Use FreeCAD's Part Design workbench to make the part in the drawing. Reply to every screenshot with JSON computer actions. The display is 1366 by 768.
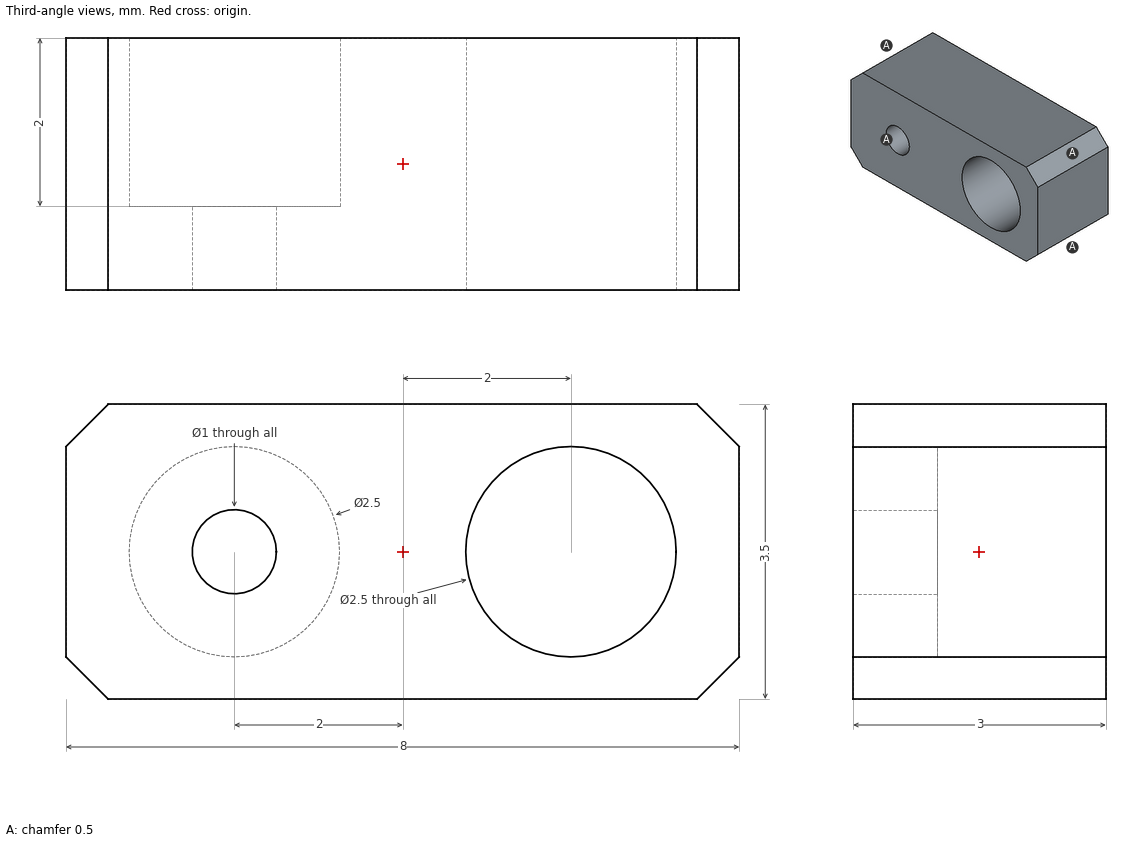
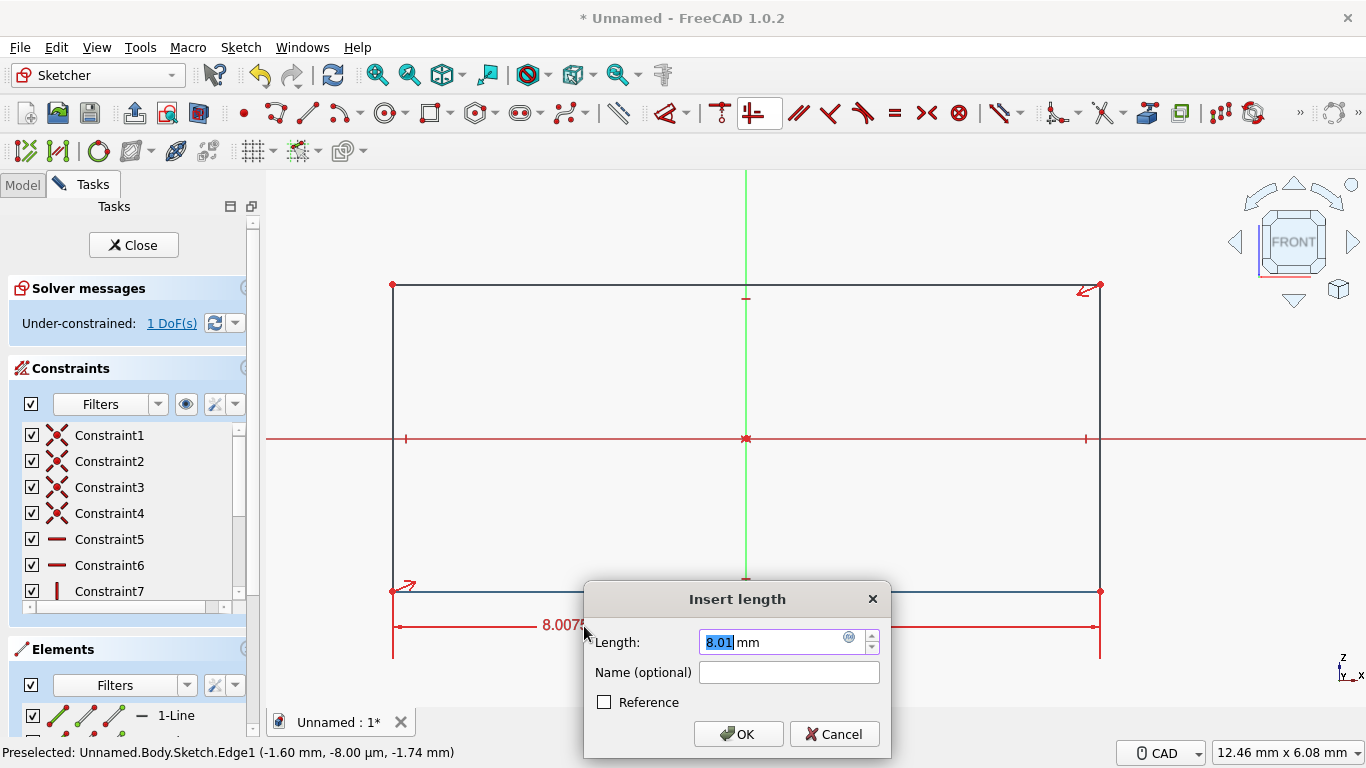
{"action": "type", "text": "8"}
{"action": "key", "text": "Return"}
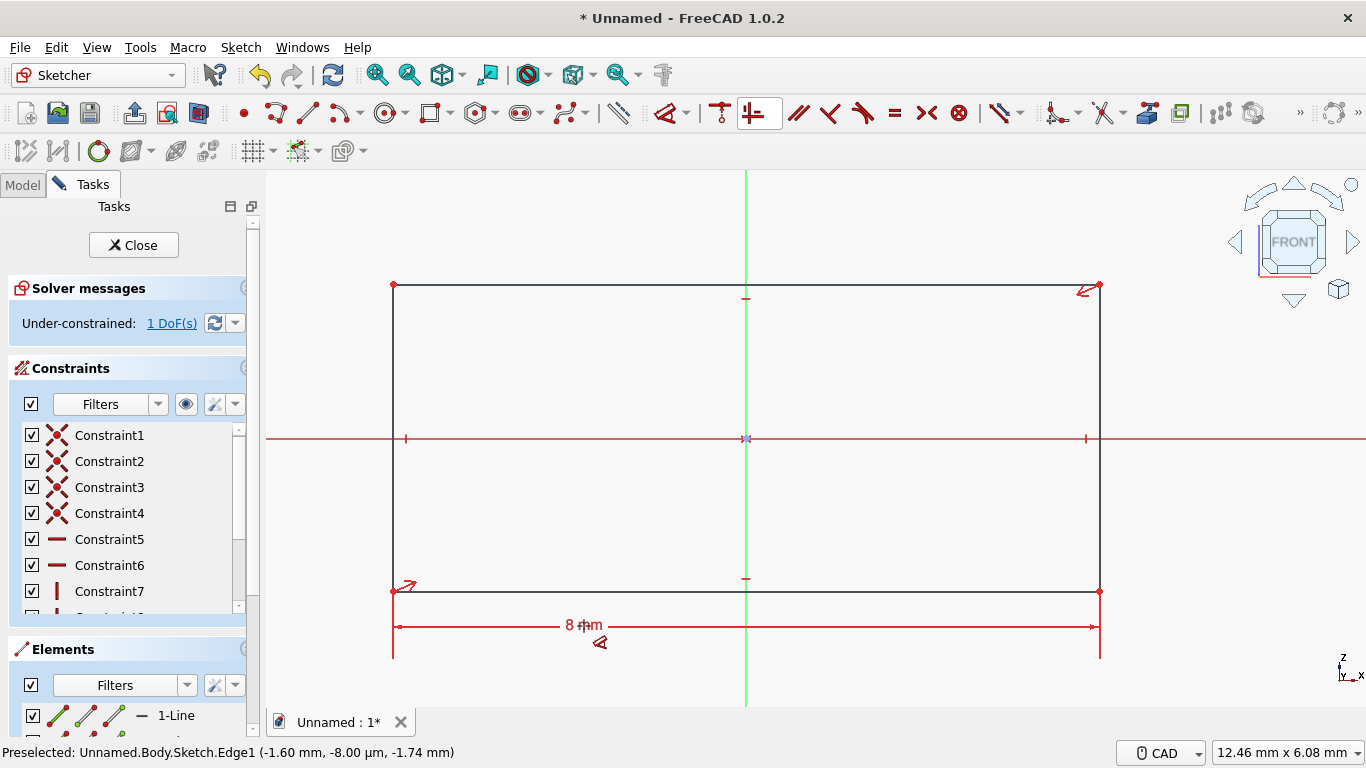
{"action": "left_click", "coordinate": [1100, 500]}
{"action": "left_click", "coordinate": [1134, 368]}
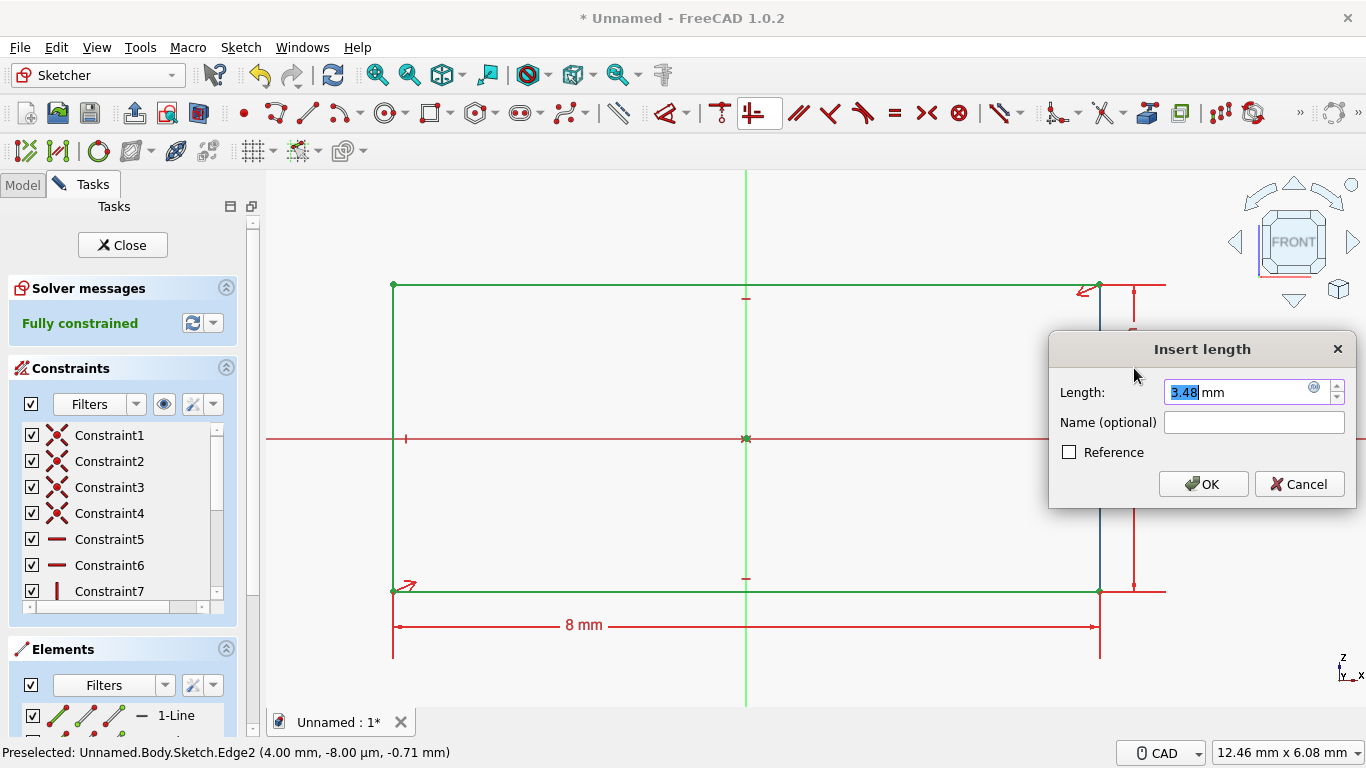
{"action": "type", "text": "3.5"}
{"action": "key", "text": "Return"}
{"action": "key", "text": "Escape"}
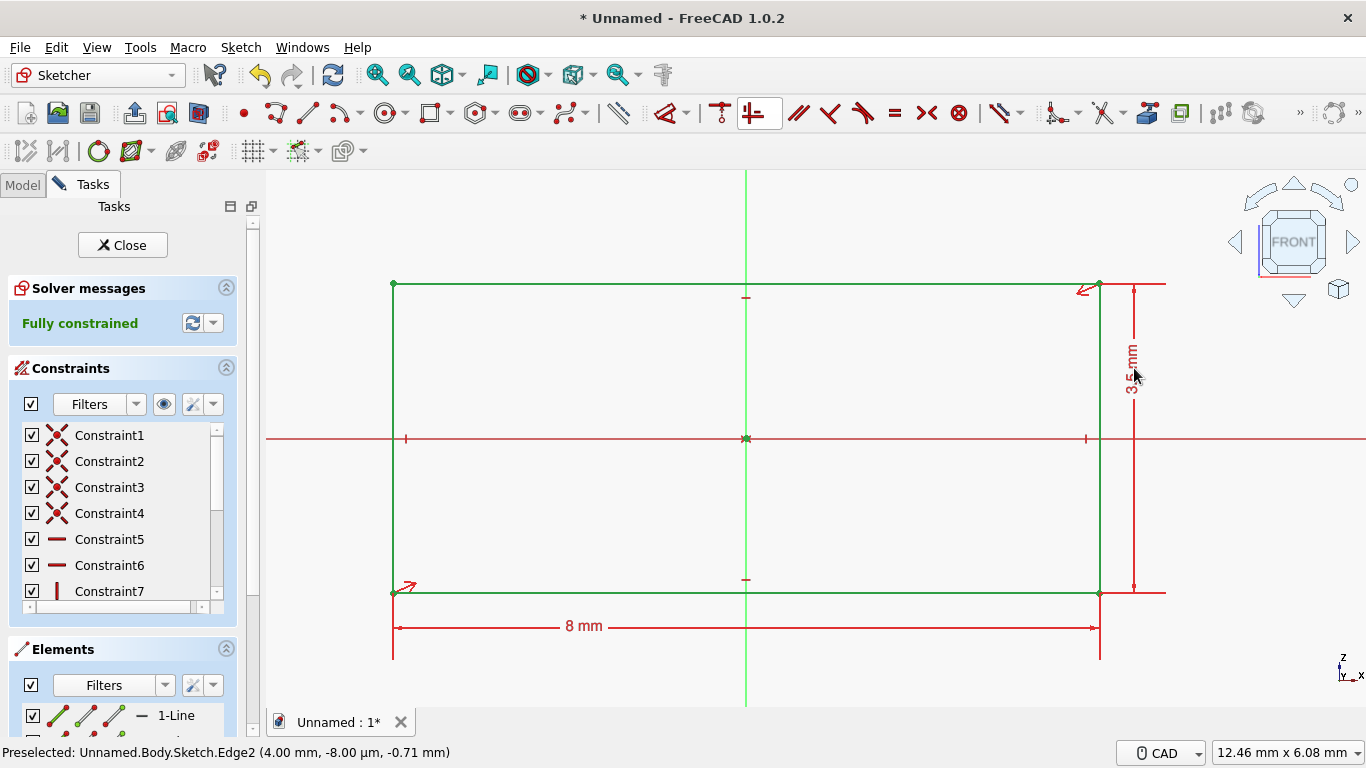
{"action": "left_click", "coordinate": [123, 245]}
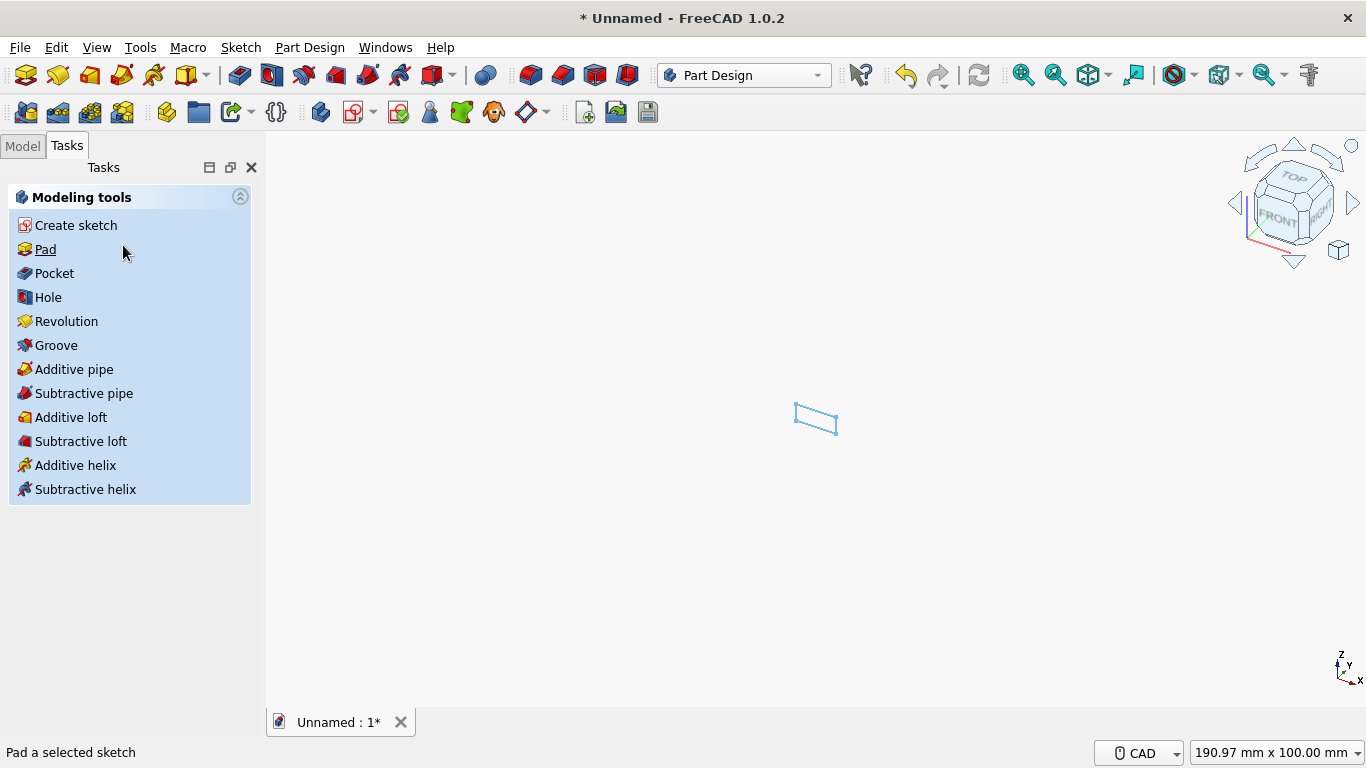
{"action": "left_click", "coordinate": [26, 76]}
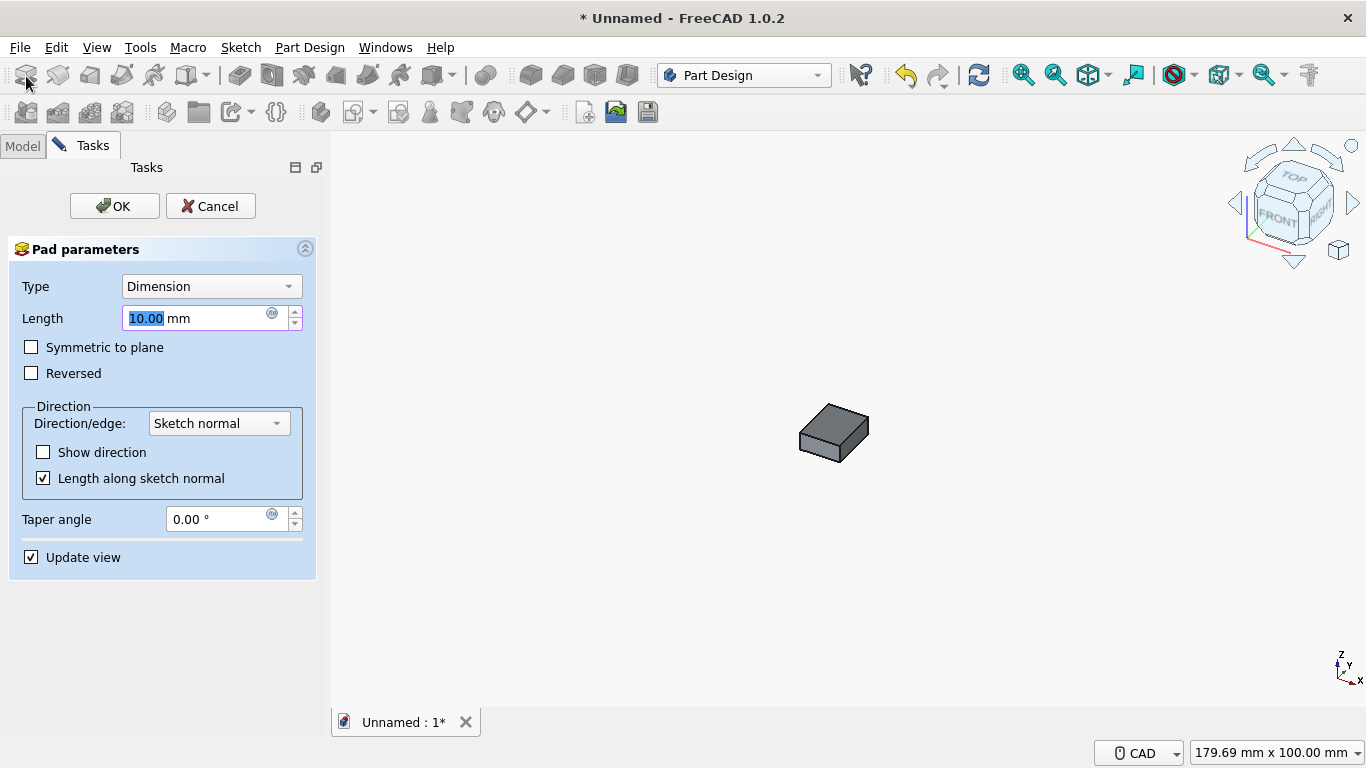
{"action": "type", "text": "3"}
{"action": "key", "text": "Tab"}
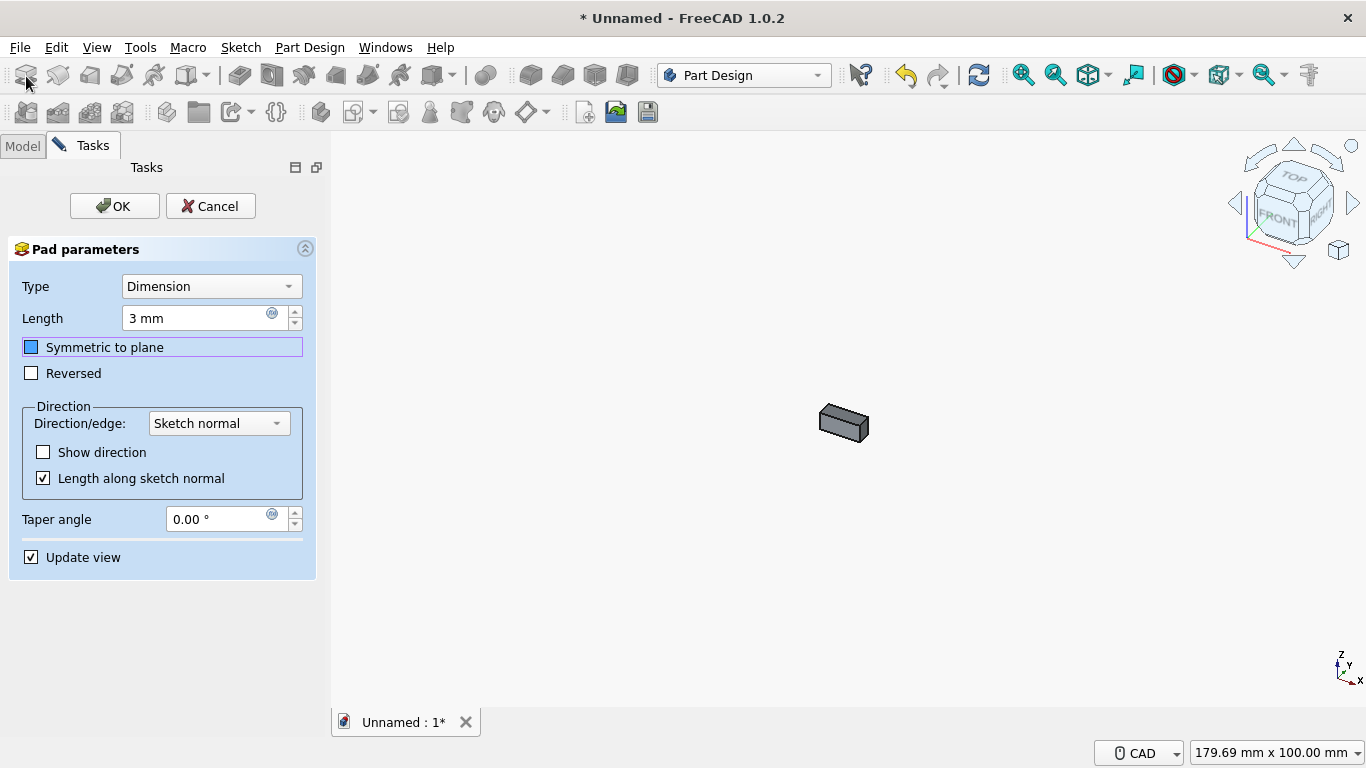
{"action": "left_click", "coordinate": [30, 347]}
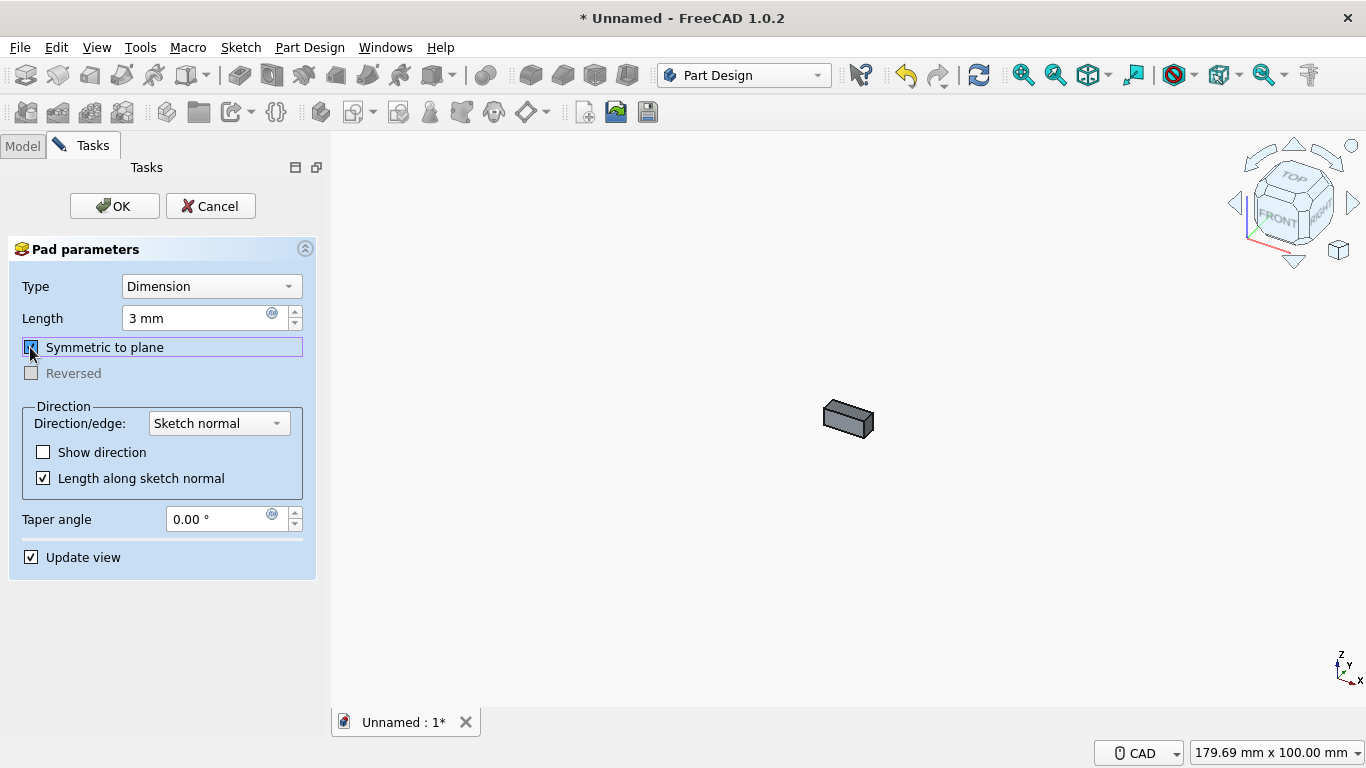
{"action": "left_click", "coordinate": [115, 206]}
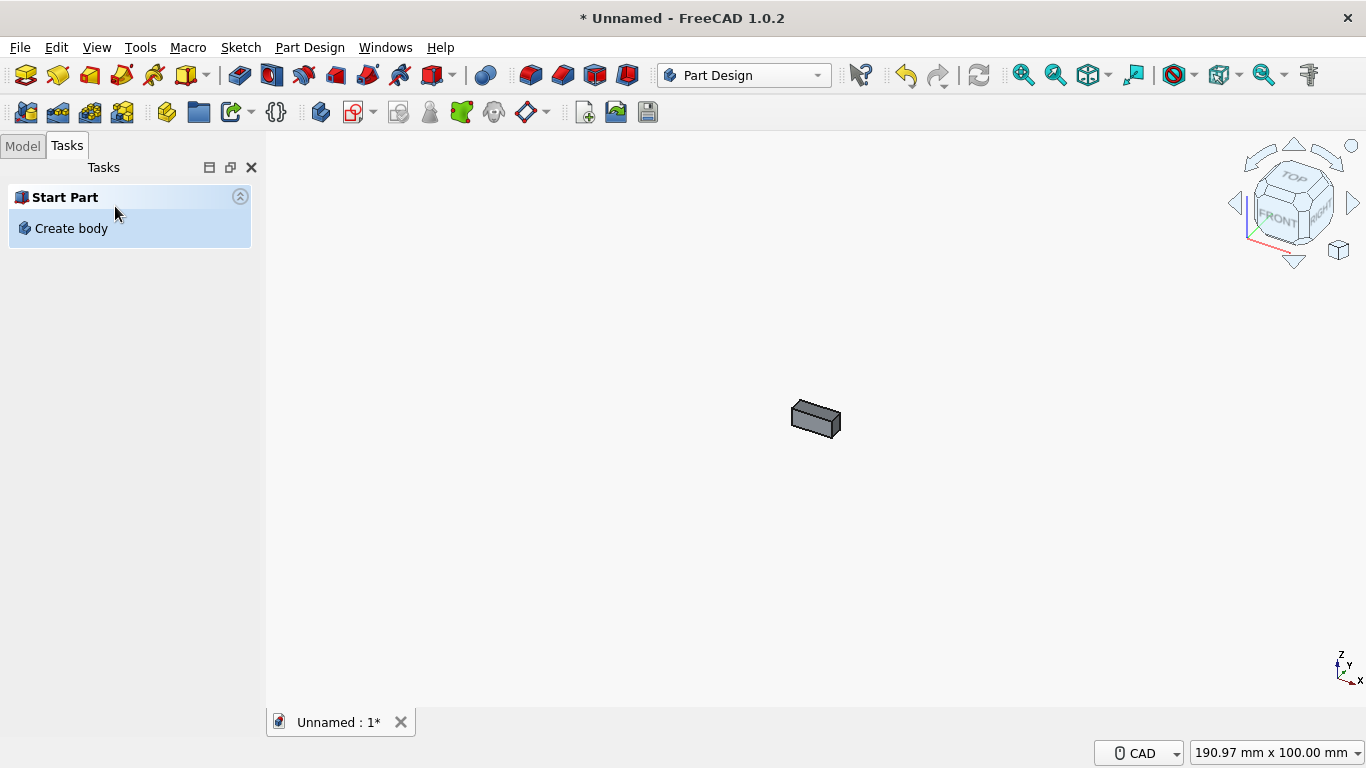
{"action": "left_click", "coordinate": [1024, 76]}